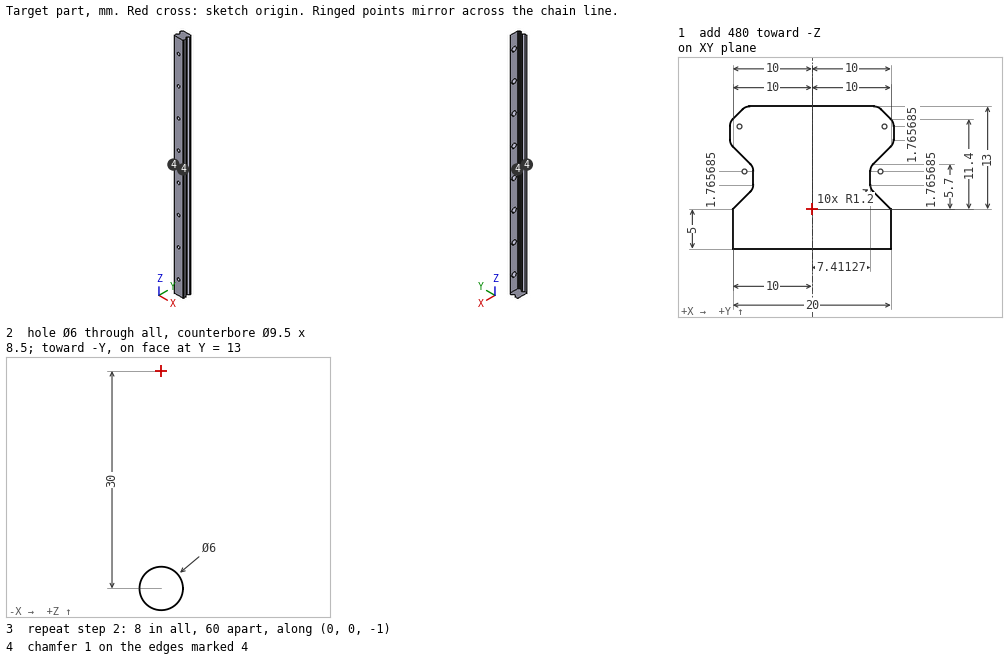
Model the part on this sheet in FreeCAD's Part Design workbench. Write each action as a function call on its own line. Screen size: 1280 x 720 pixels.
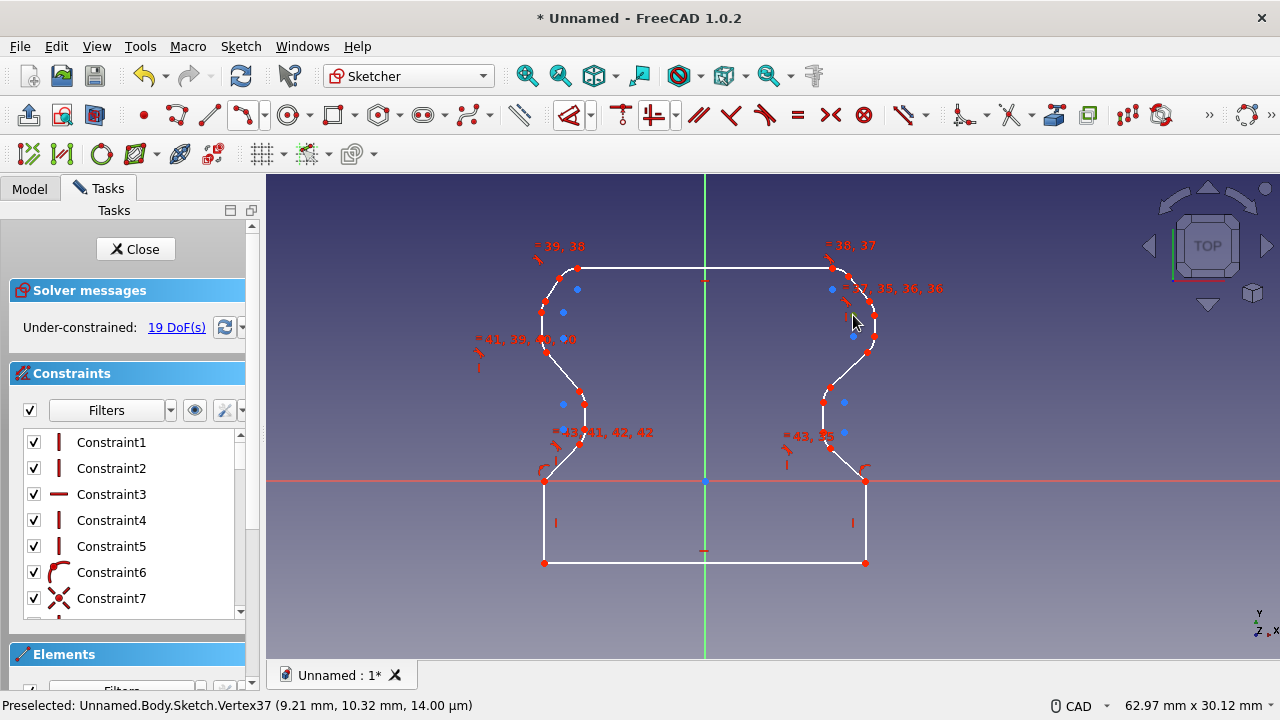
click(563, 312)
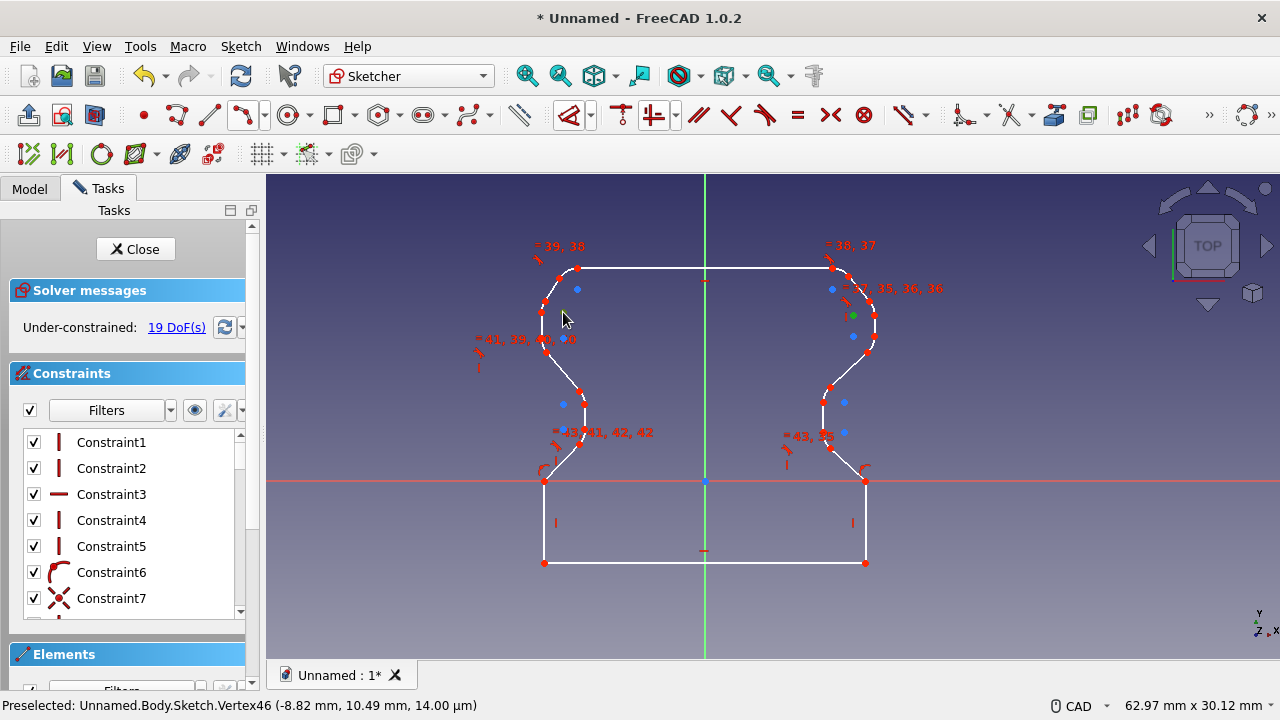
click(705, 600)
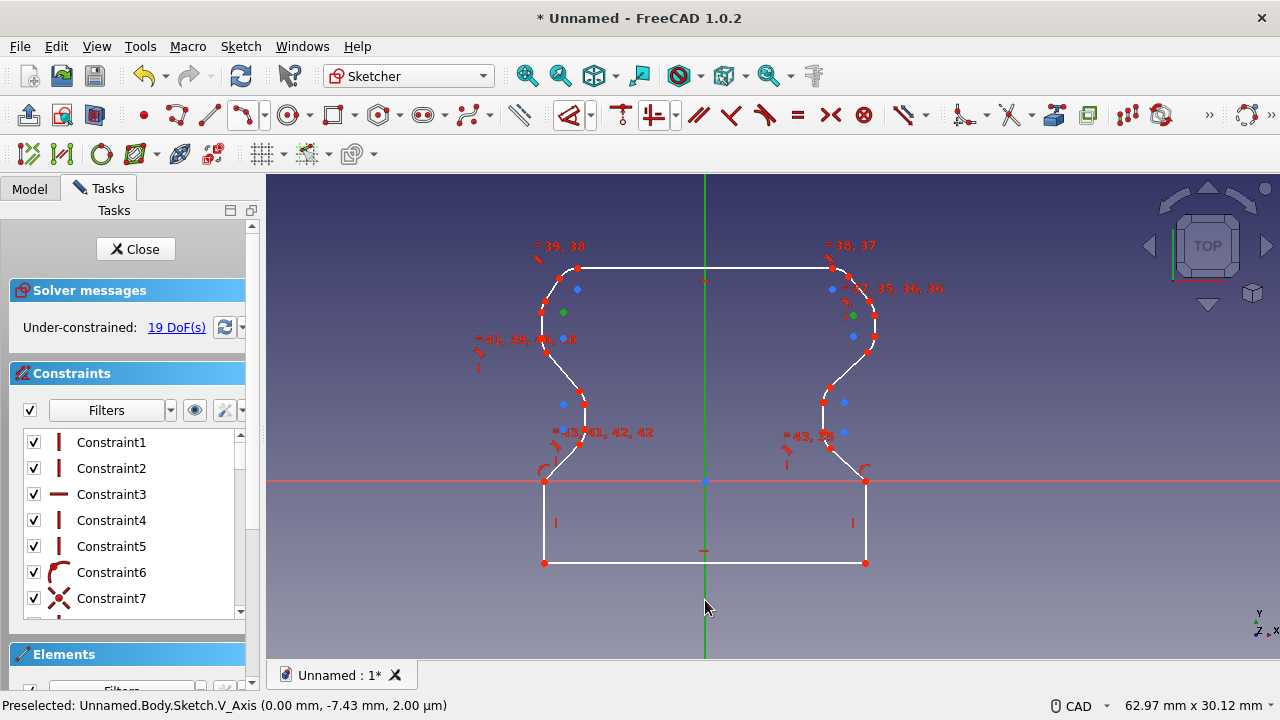
key(s)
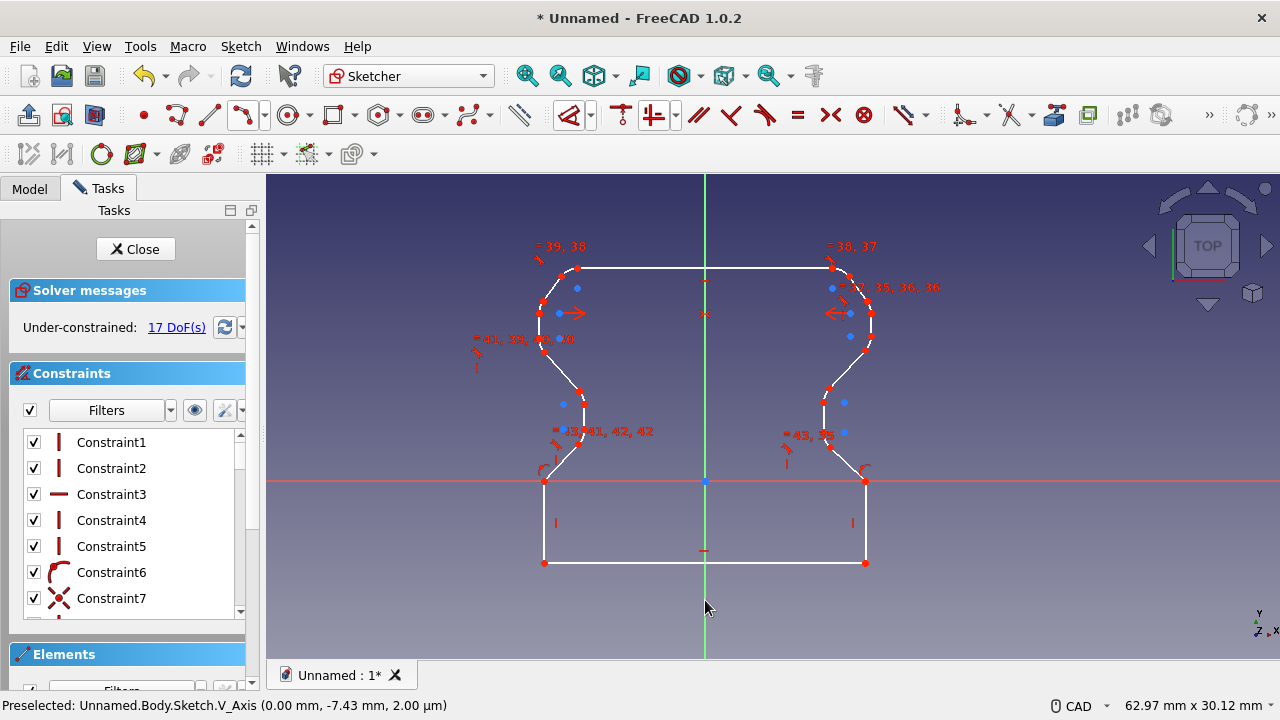
click(845, 403)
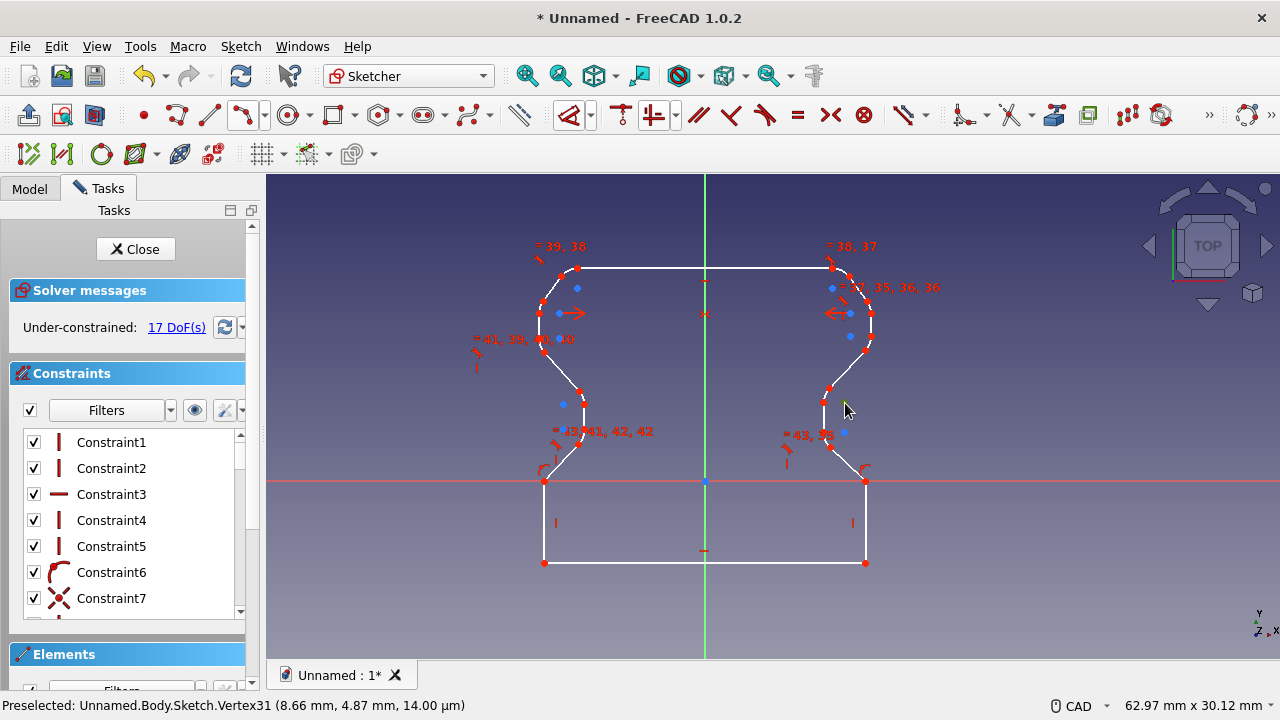
click(564, 405)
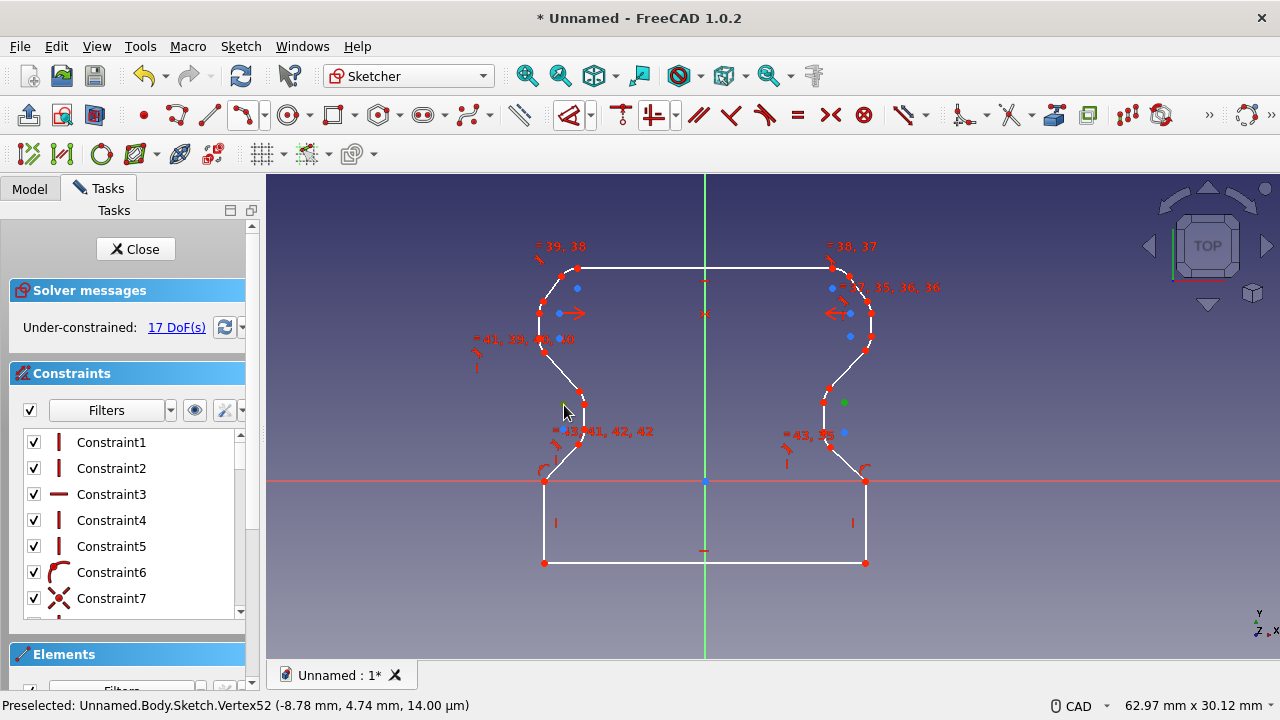
click(705, 600)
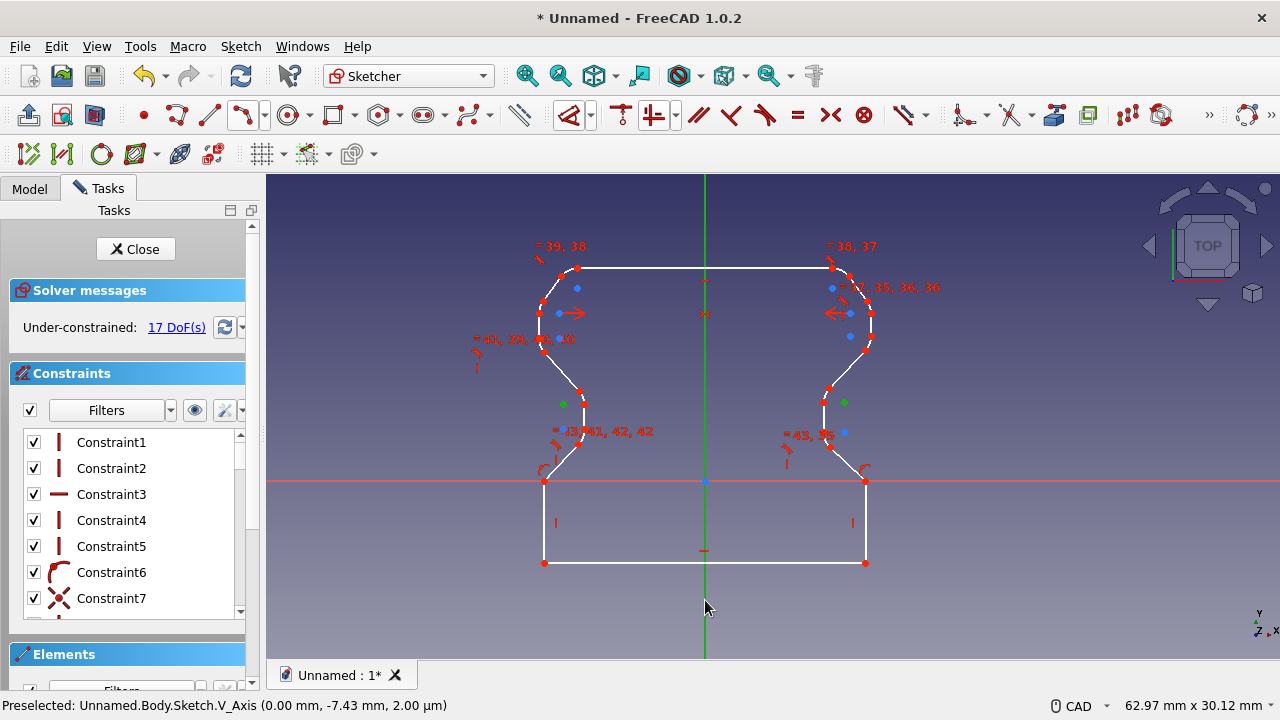
click(831, 116)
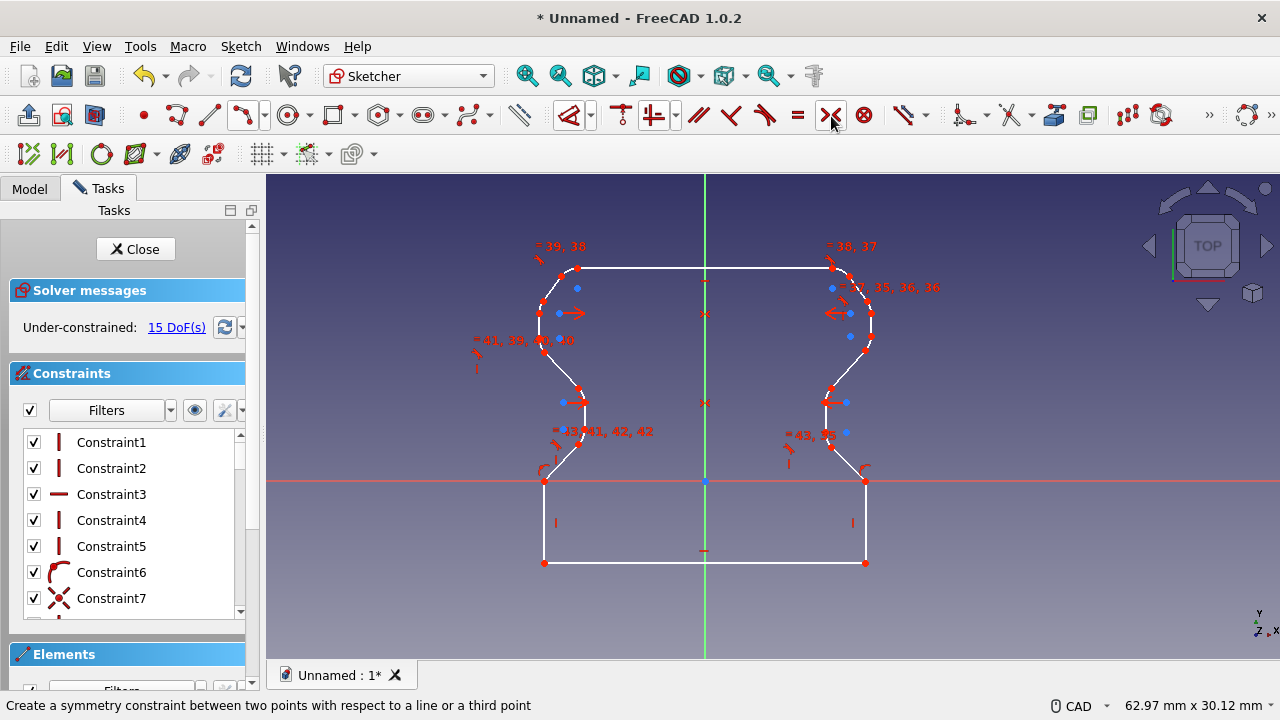
key(d)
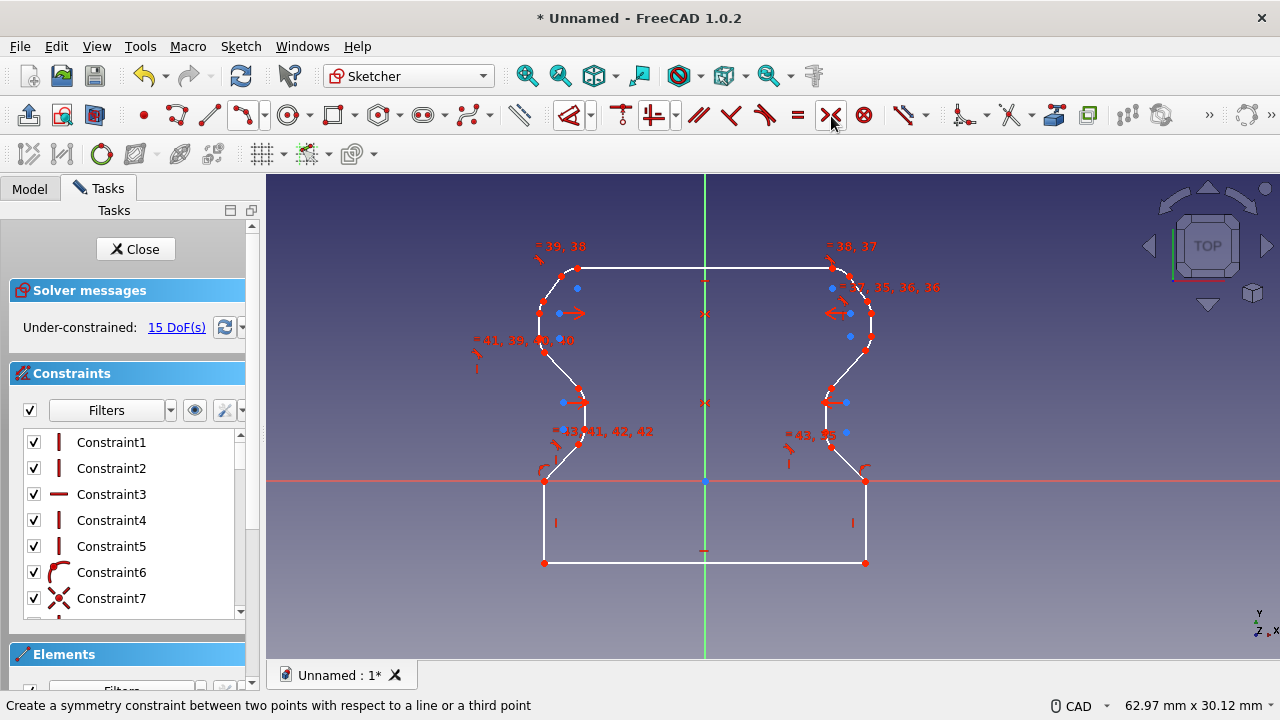
scroll(827, 395, up, 4)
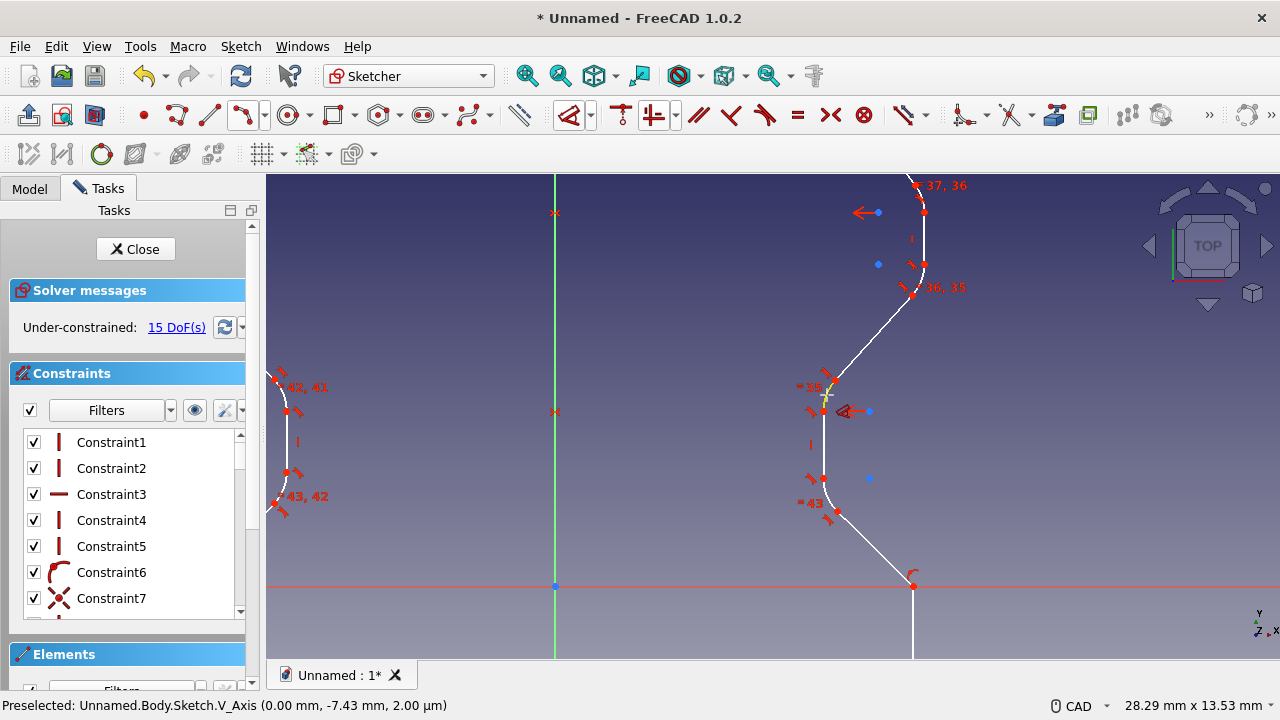
click(827, 395)
click(797, 384)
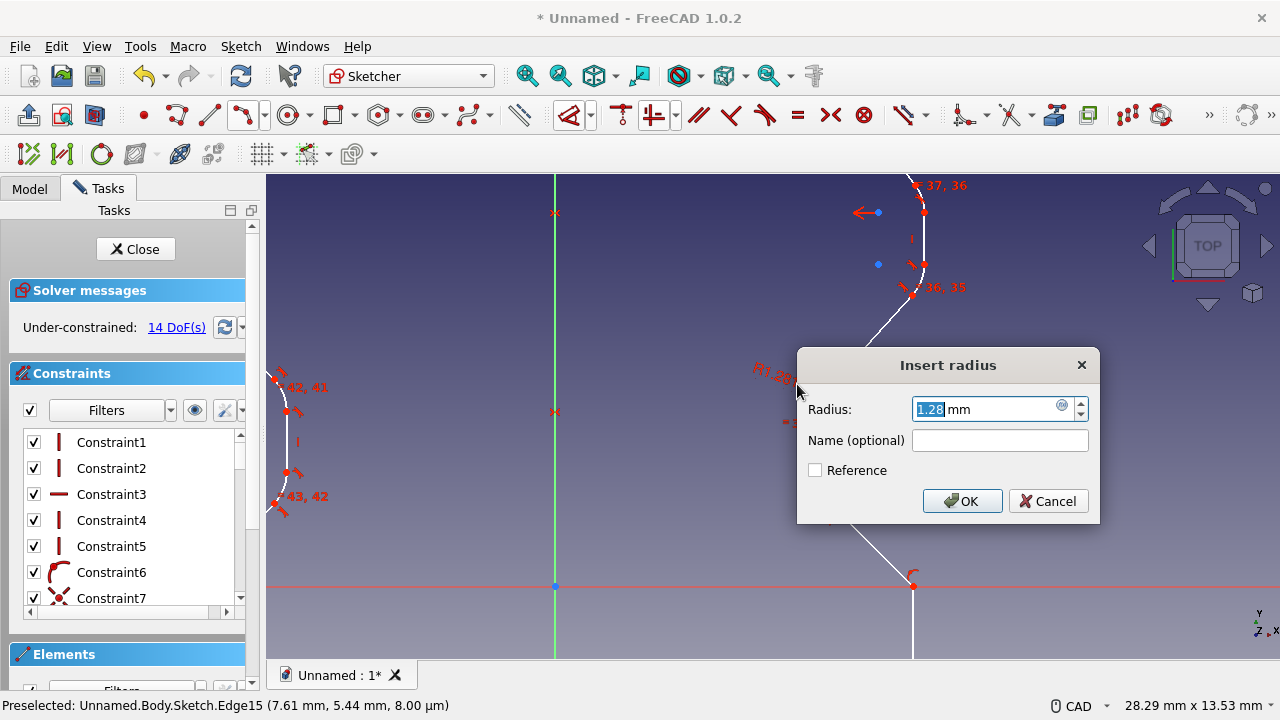
text(1.2)
key(Return)